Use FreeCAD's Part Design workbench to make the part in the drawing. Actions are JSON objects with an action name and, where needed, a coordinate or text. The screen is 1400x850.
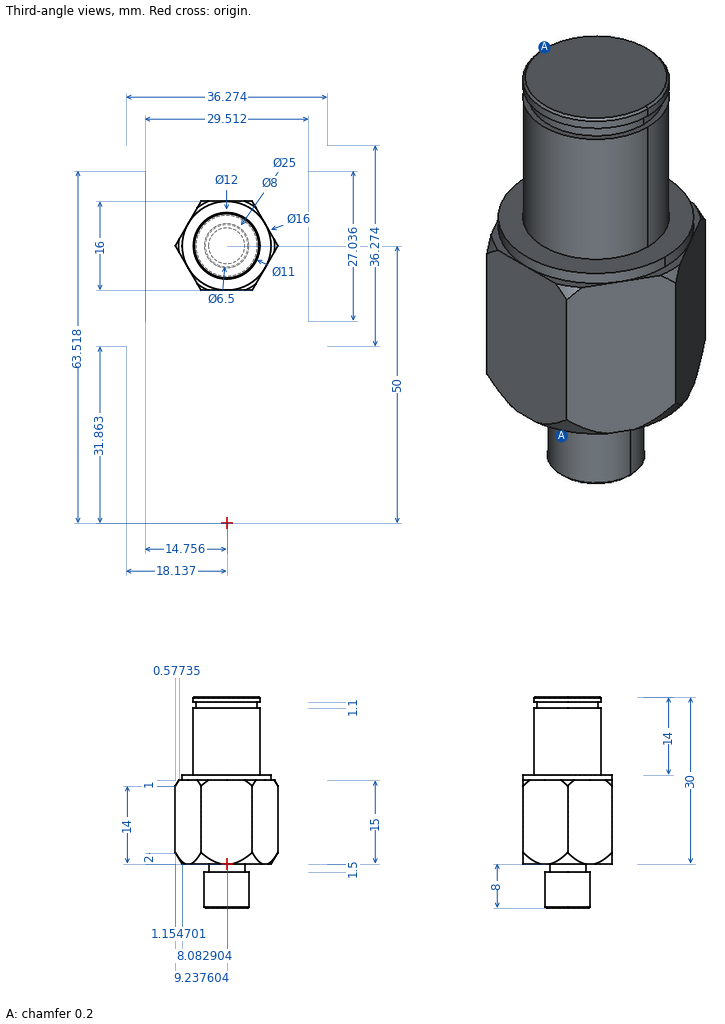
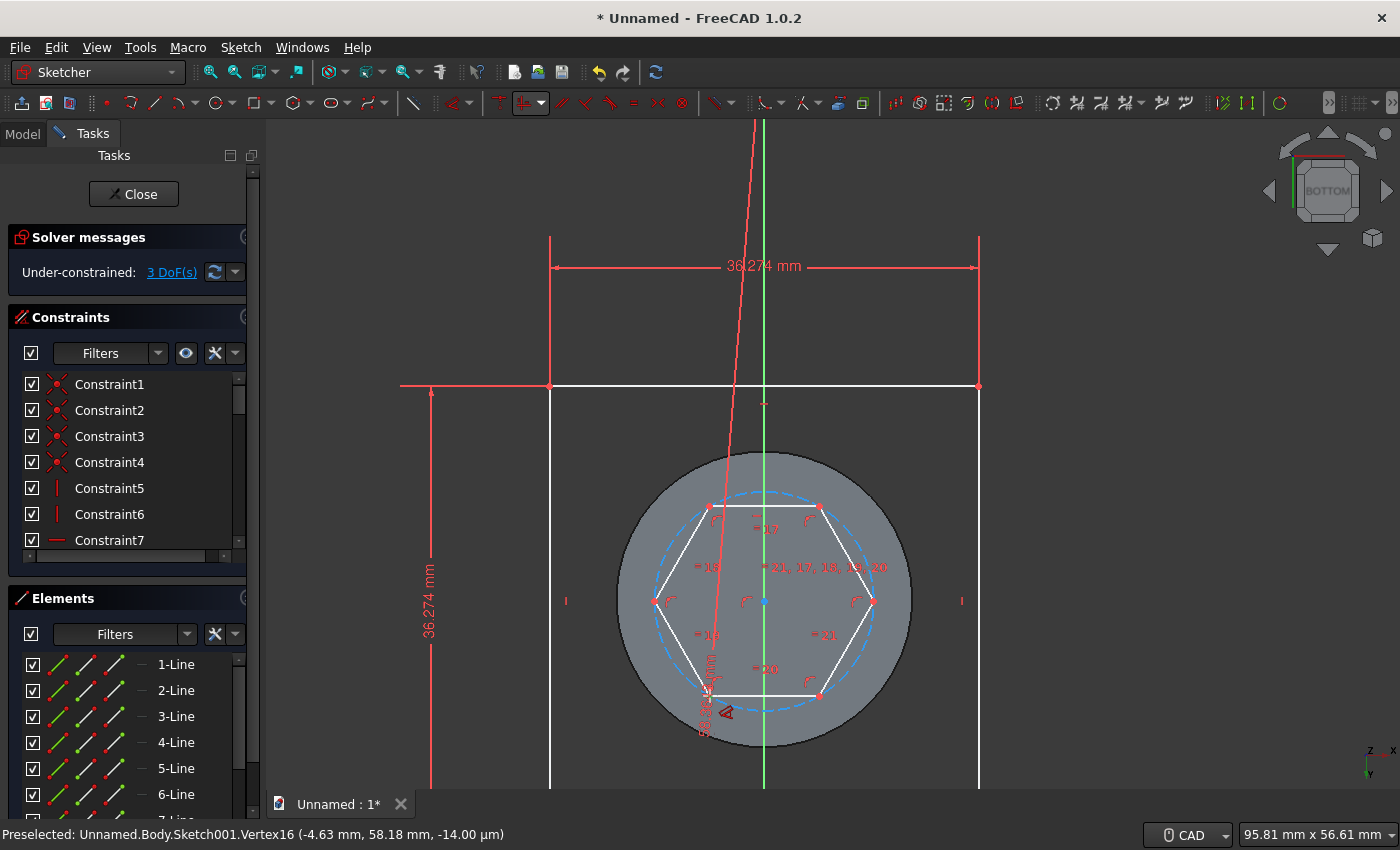
{"action": "left_click", "coordinate": [819, 506]}
{"action": "left_click", "coordinate": [853, 601]}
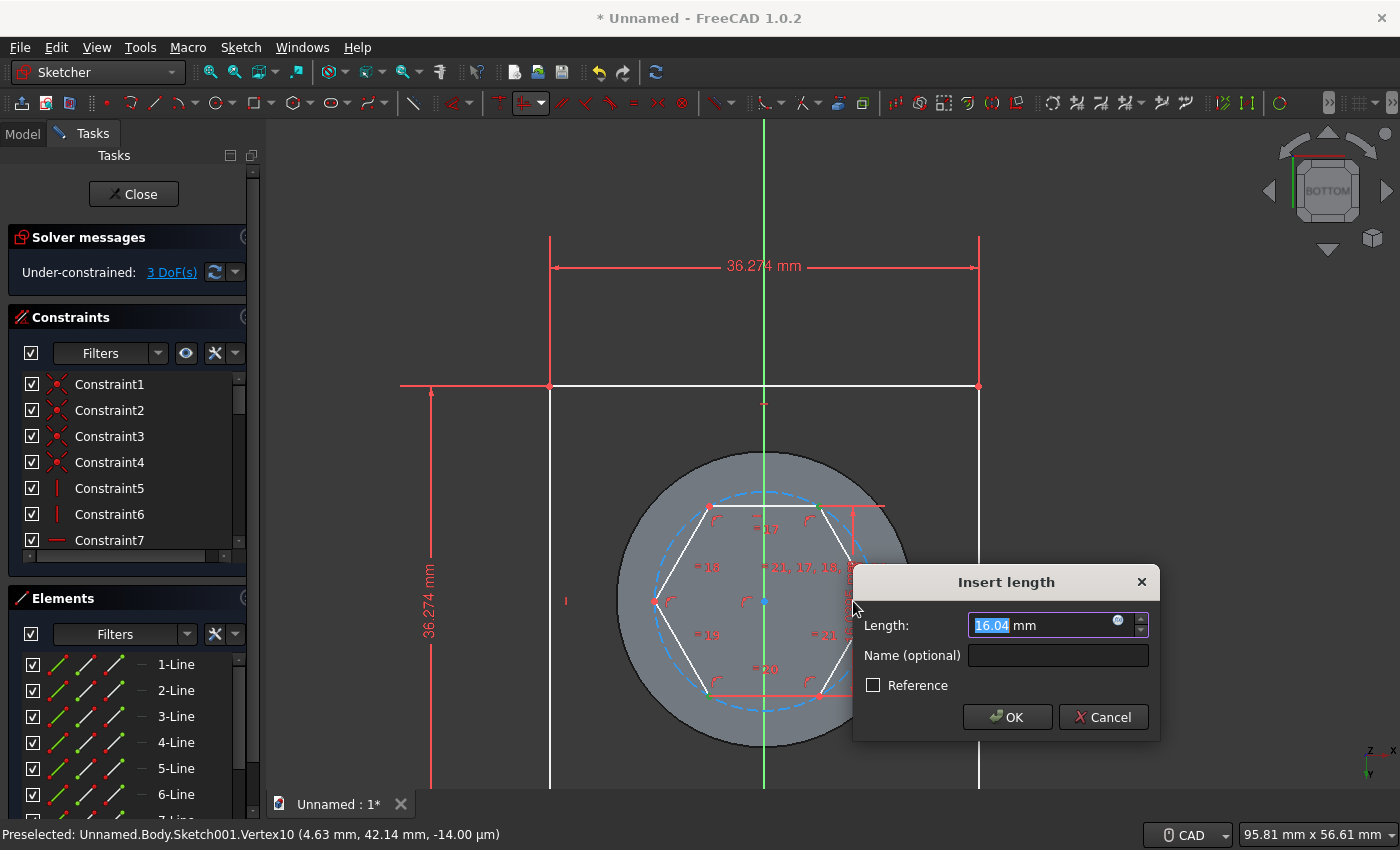
{"action": "type", "text": "16"}
{"action": "key", "text": "Return"}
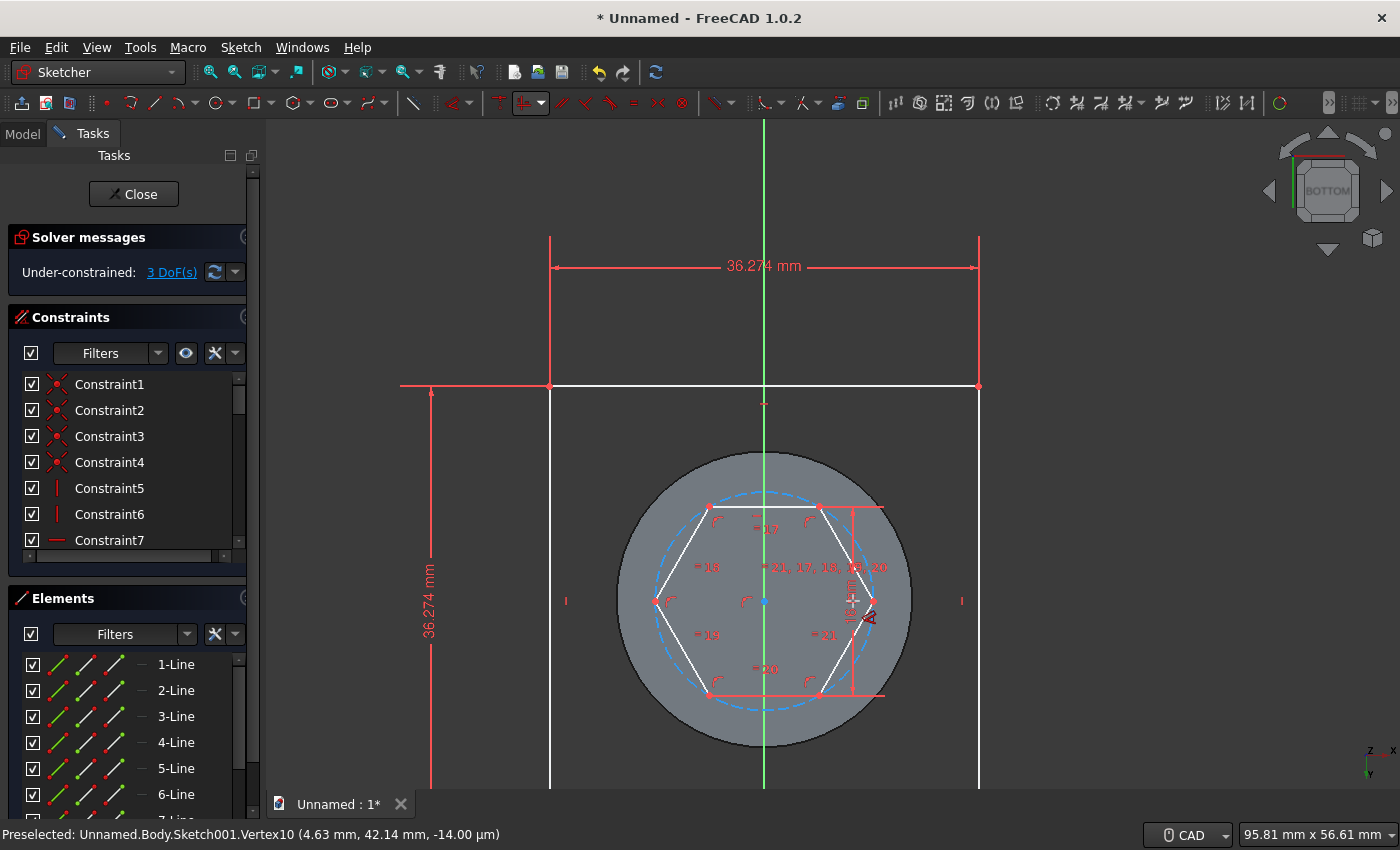
{"action": "left_click", "coordinate": [764, 601]}
{"action": "left_click", "coordinate": [798, 270]}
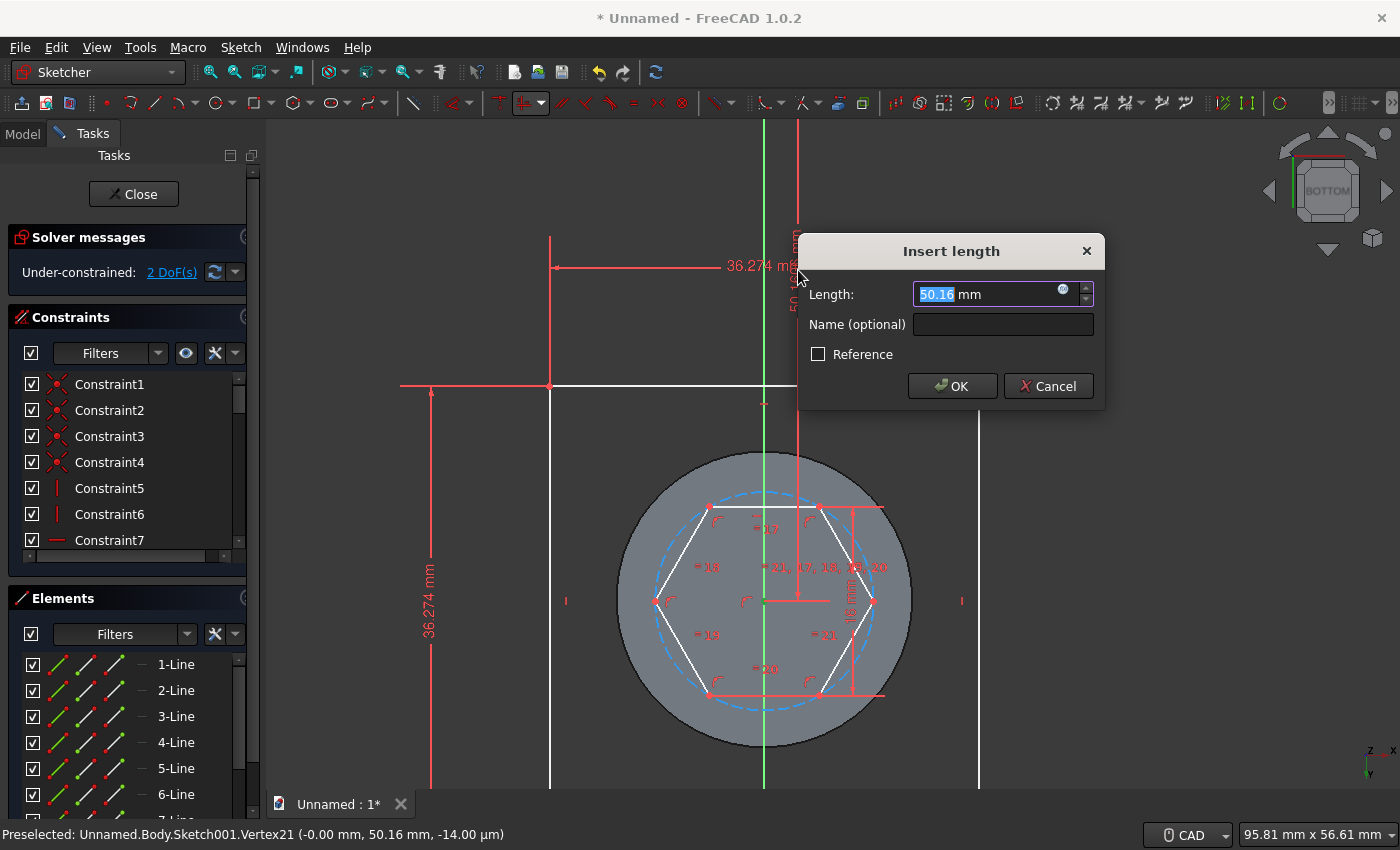
{"action": "type", "text": "50"}
{"action": "key", "text": "Return"}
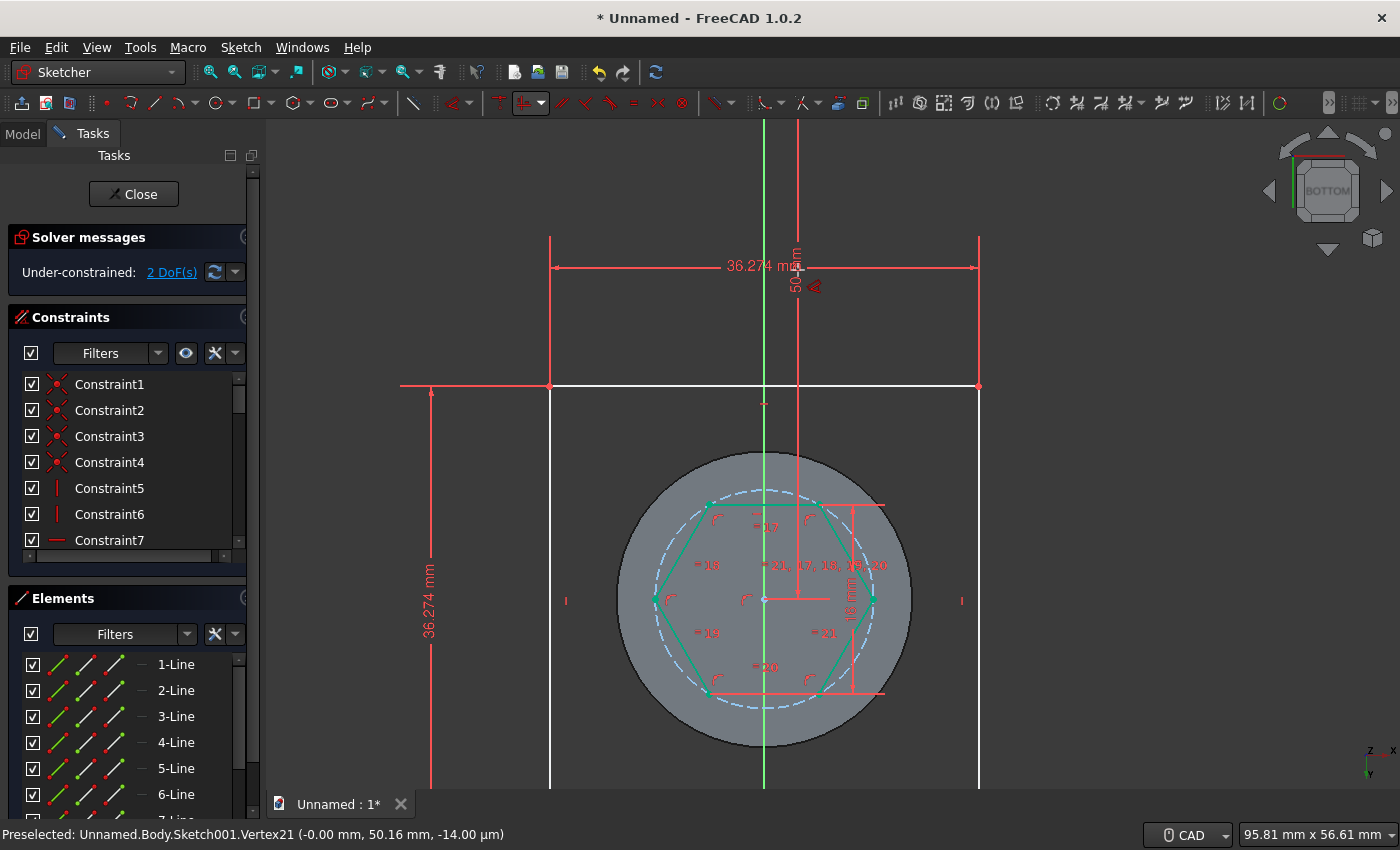
{"action": "left_click", "coordinate": [550, 386]}
{"action": "left_click", "coordinate": [657, 420]}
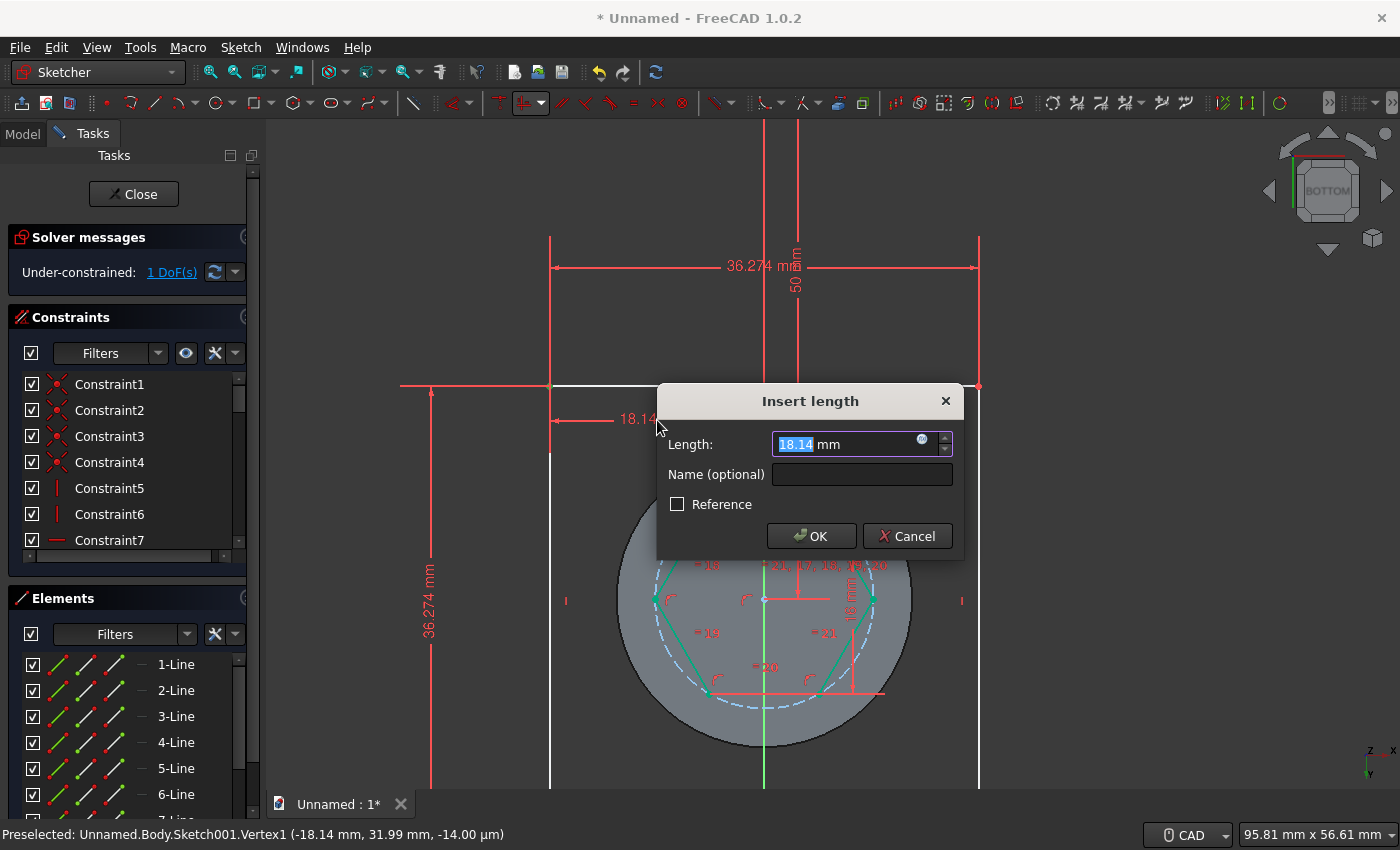
{"action": "type", "text": "18.137"}
{"action": "key", "text": "Return"}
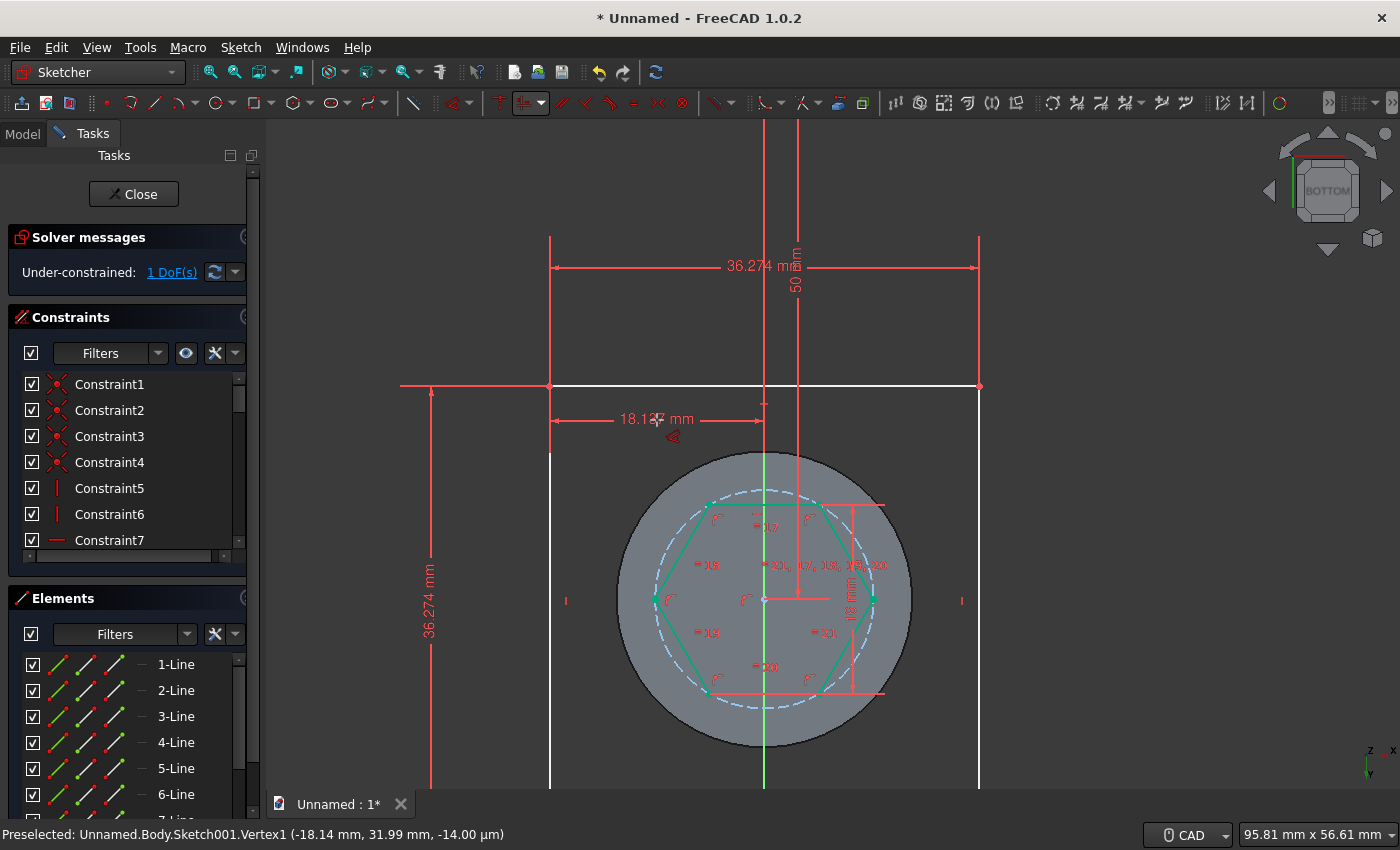
{"action": "left_click", "coordinate": [550, 386]}
{"action": "left_click", "coordinate": [516, 267]}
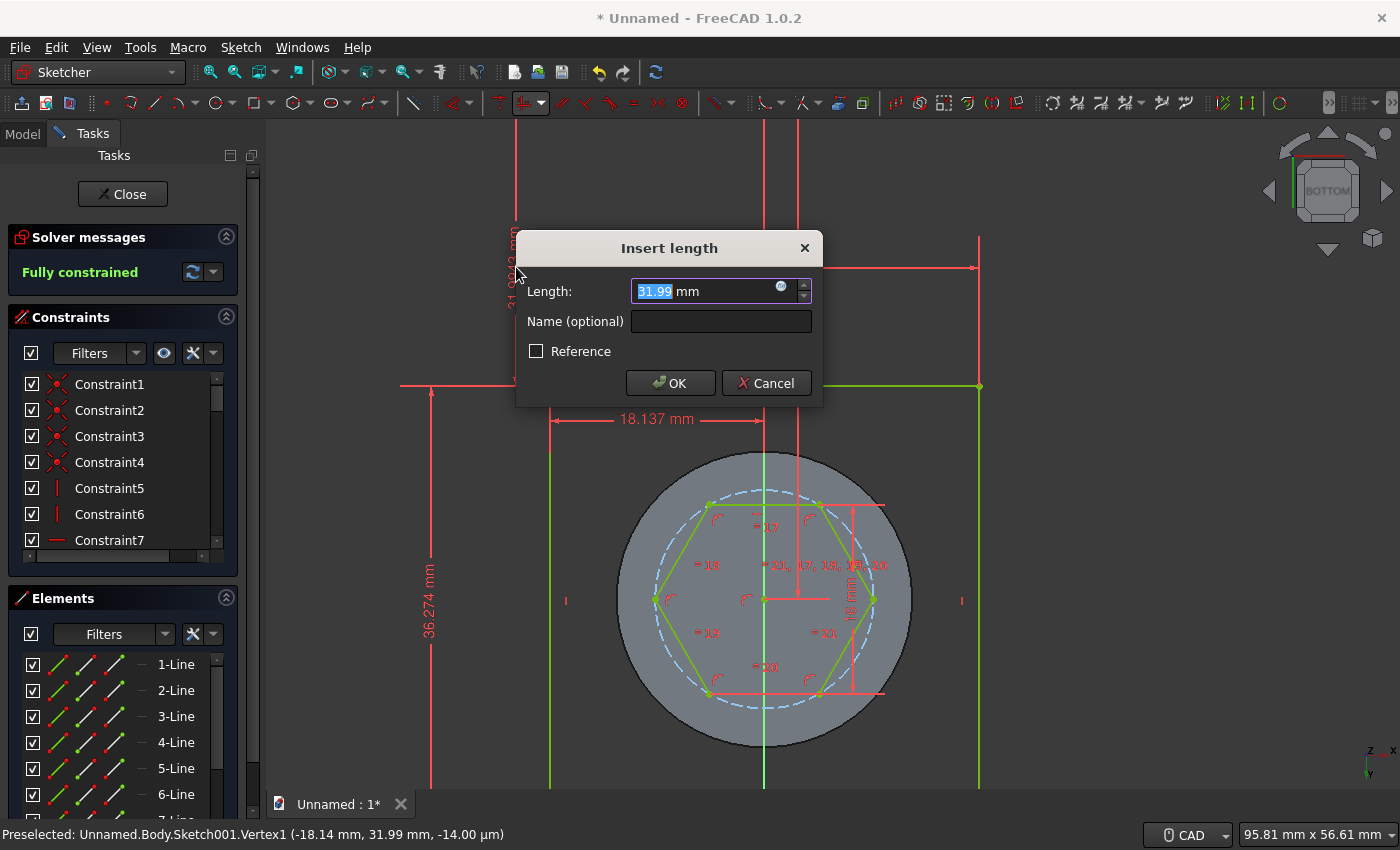
{"action": "type", "text": "31.863"}
{"action": "key", "text": "Return"}
{"action": "key", "text": "Escape"}